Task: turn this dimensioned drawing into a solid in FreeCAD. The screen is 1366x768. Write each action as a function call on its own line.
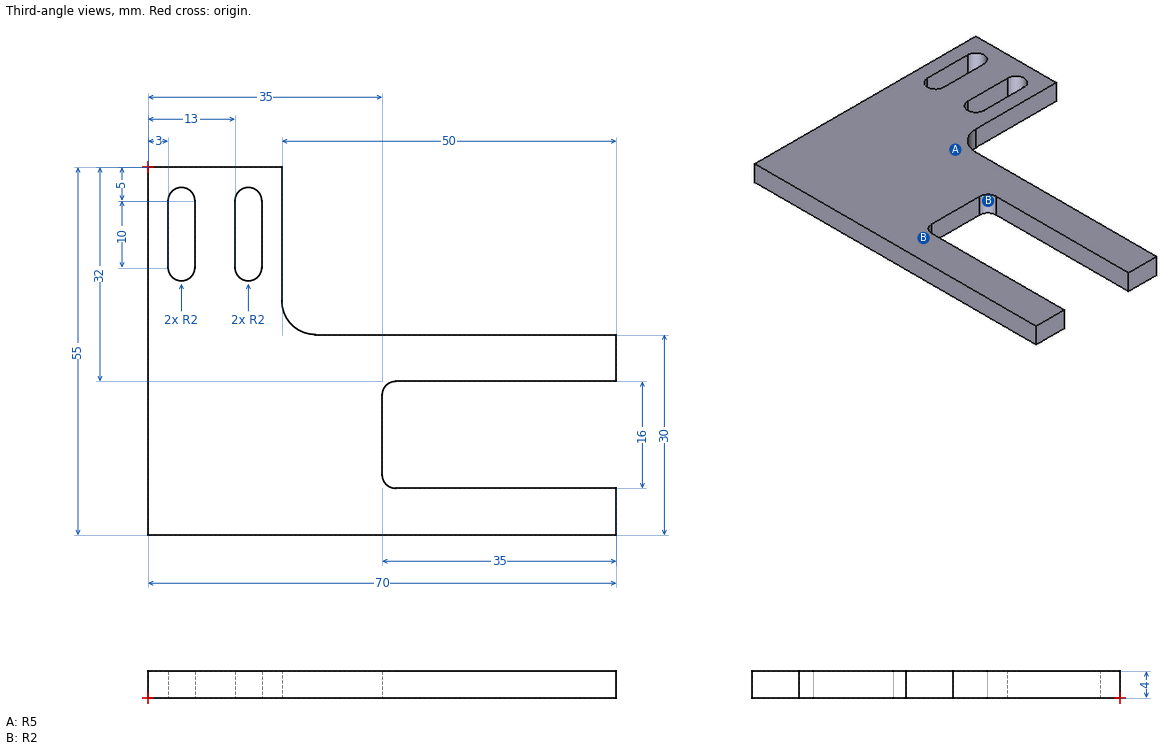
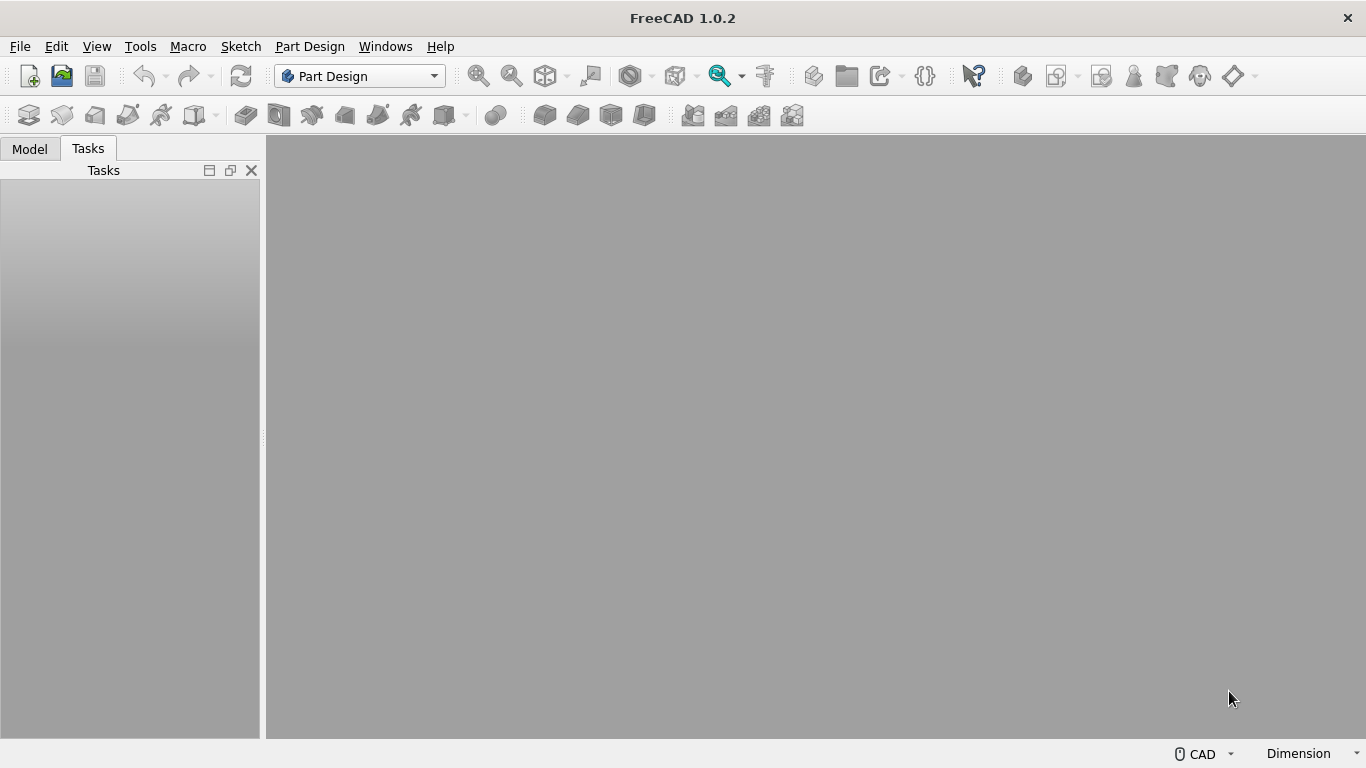
click(29, 76)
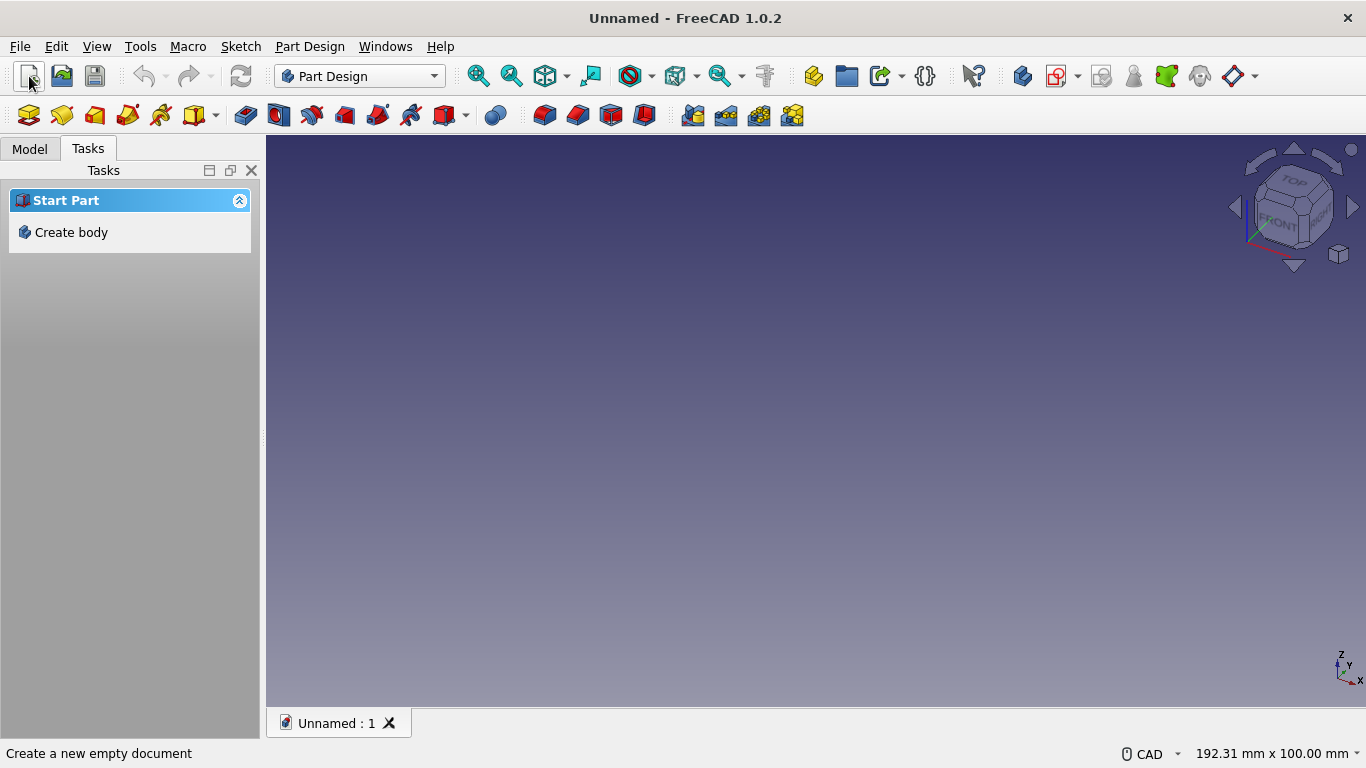
click(1056, 76)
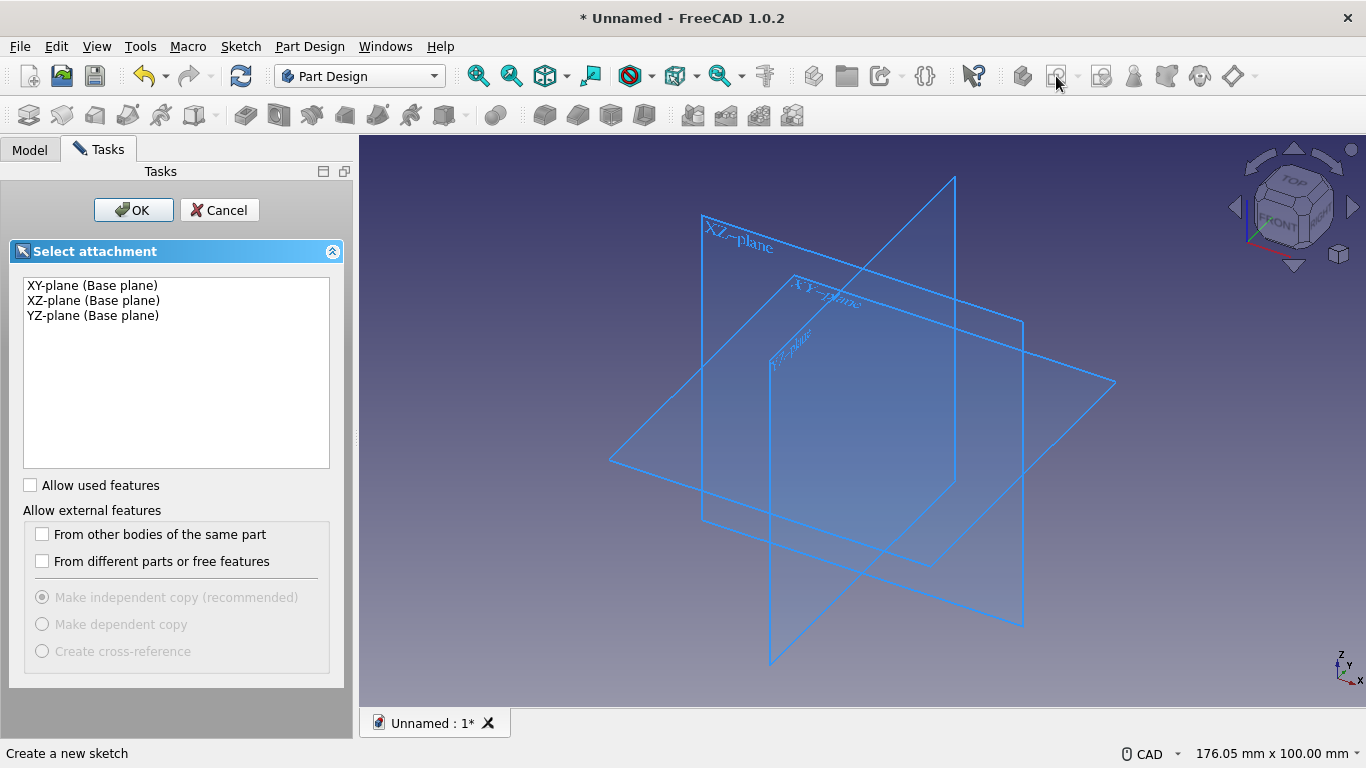
click(84, 286)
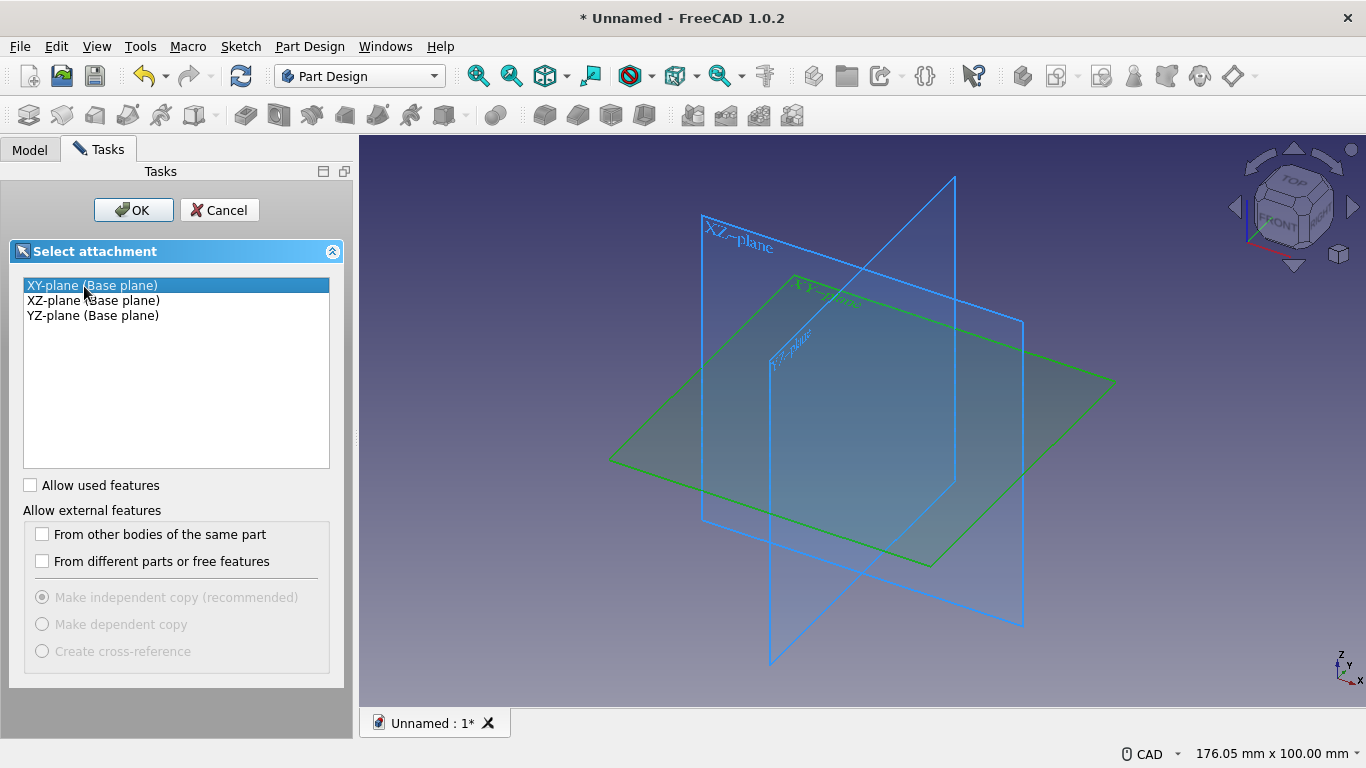
click(134, 210)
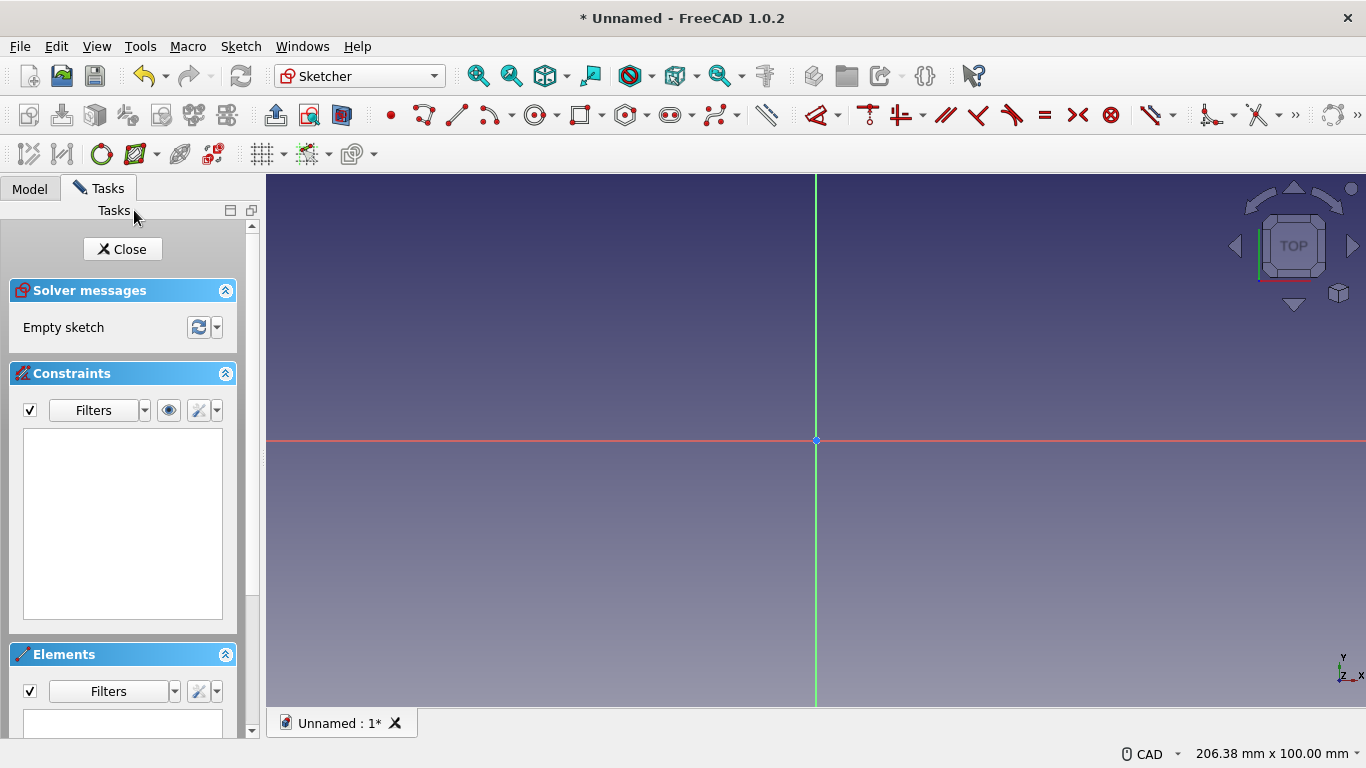
scroll(294, 202, down, 1)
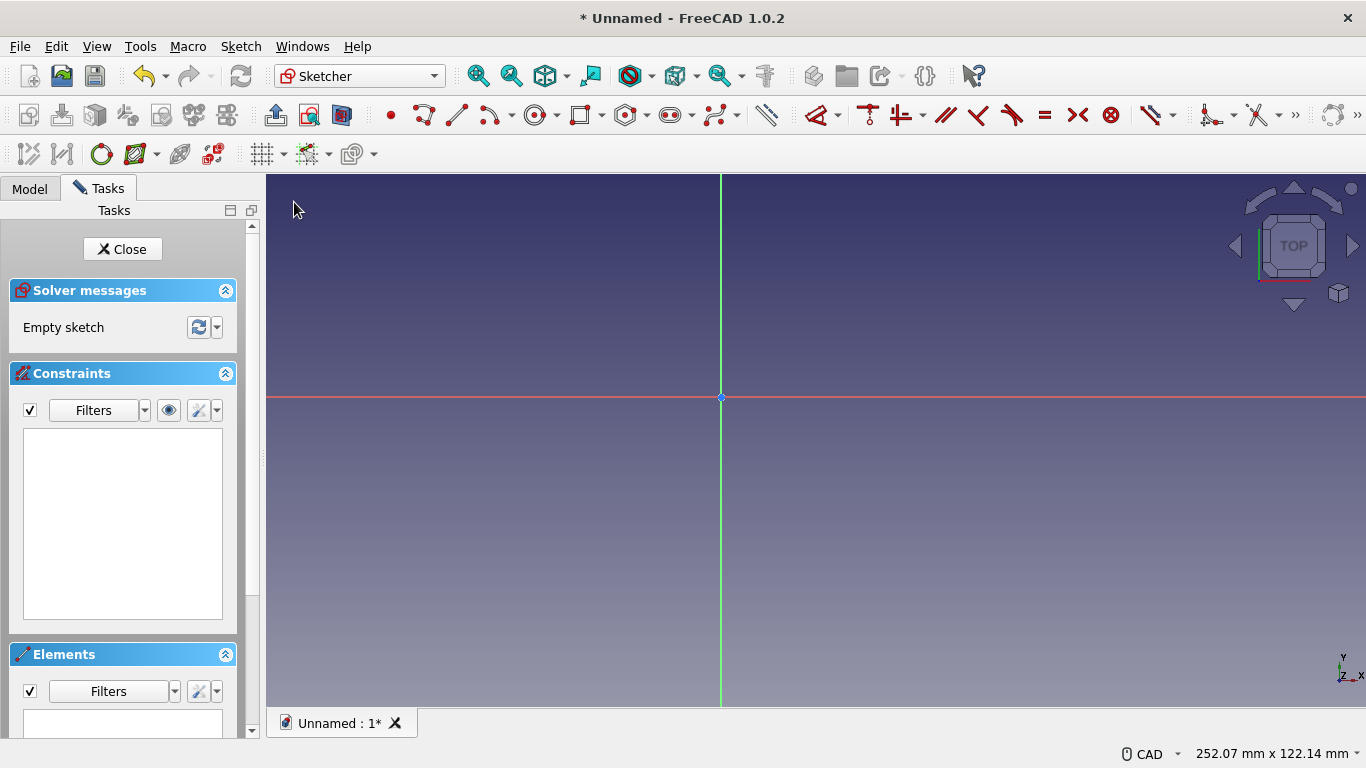
scroll(1132, 673, up, 2)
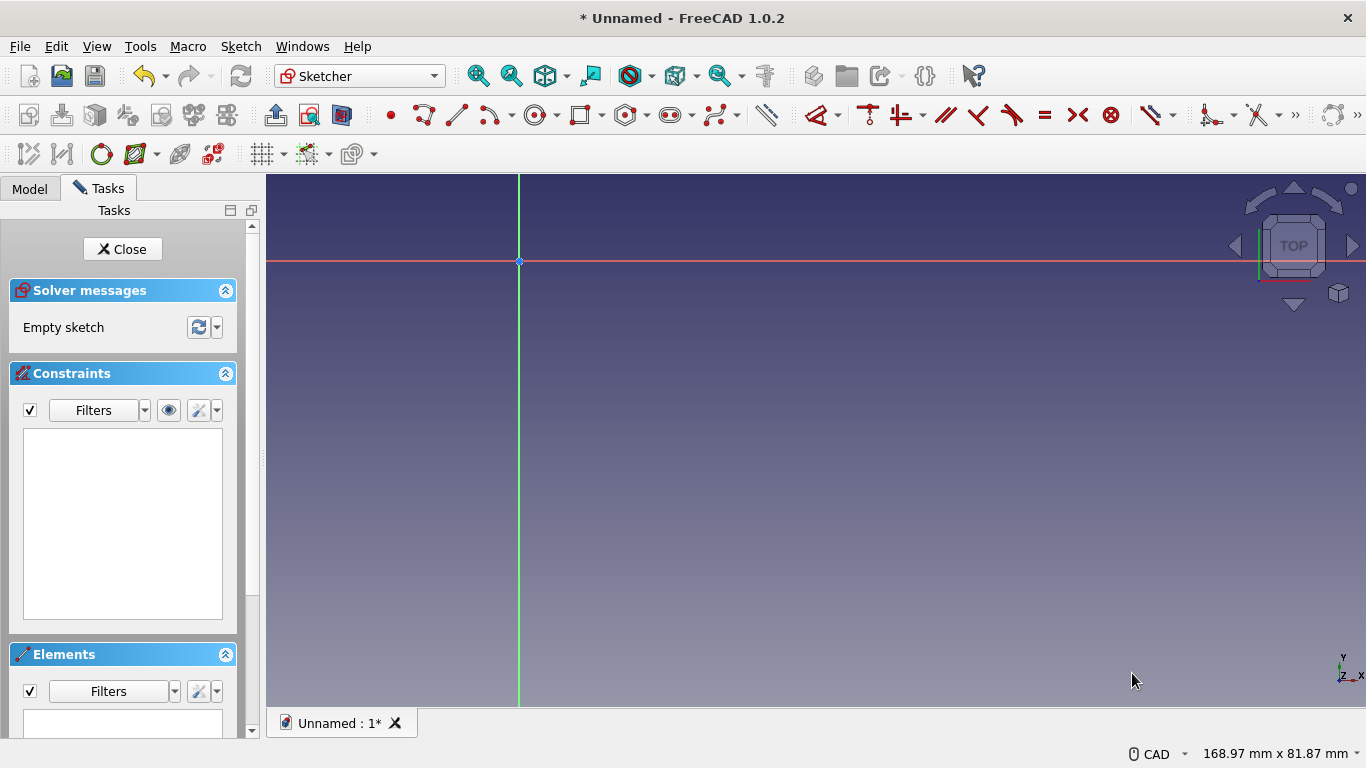
key(g)
key(m)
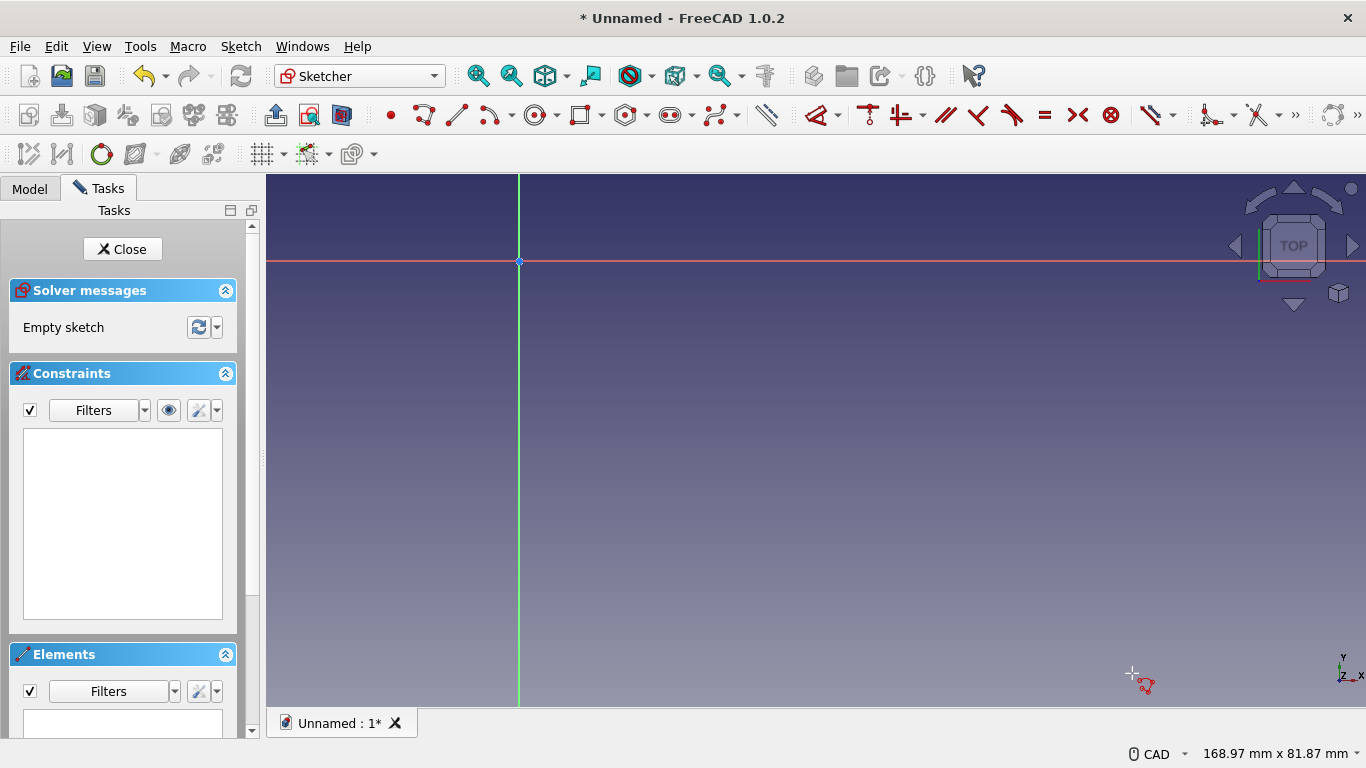
click(519, 261)
click(528, 619)
click(975, 619)
click(975, 424)
click(649, 424)
click(649, 270)
click(519, 261)
key(Escape)
key(Escape)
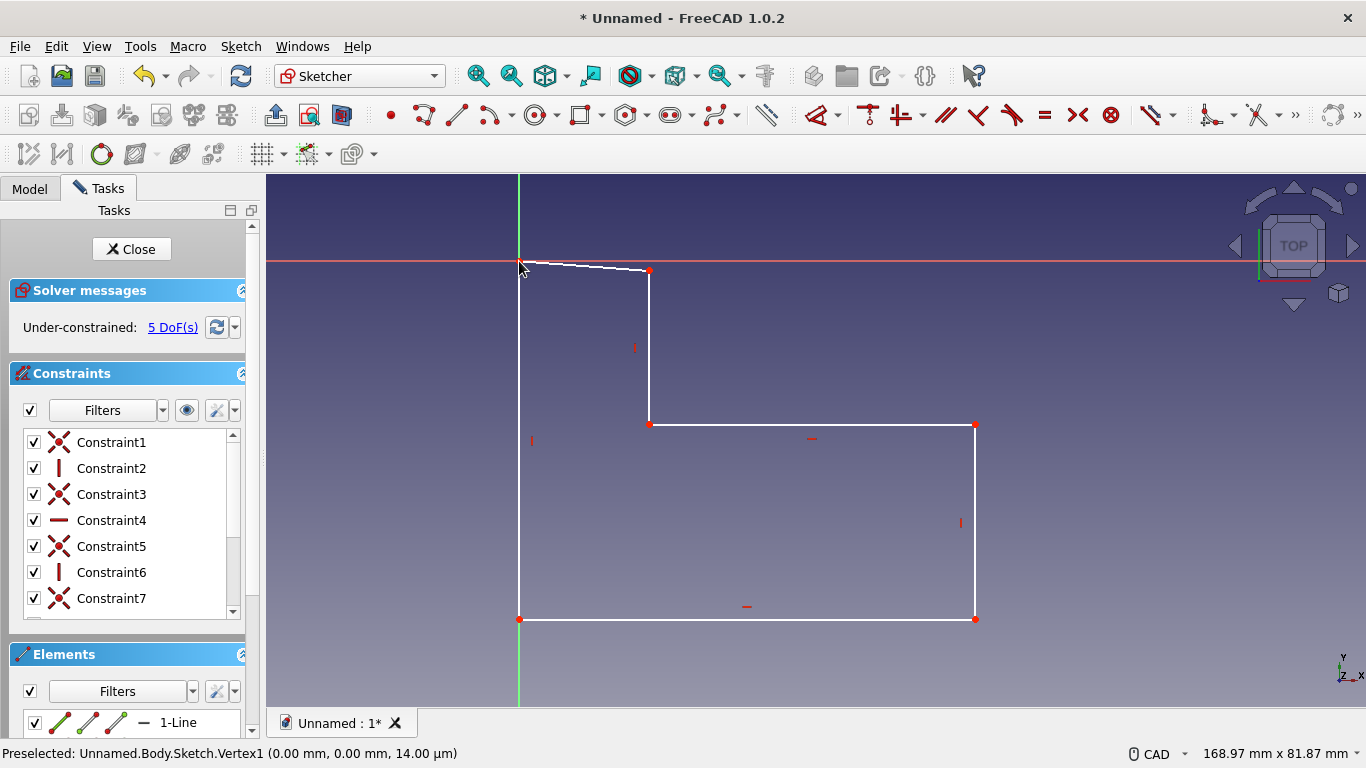
click(558, 264)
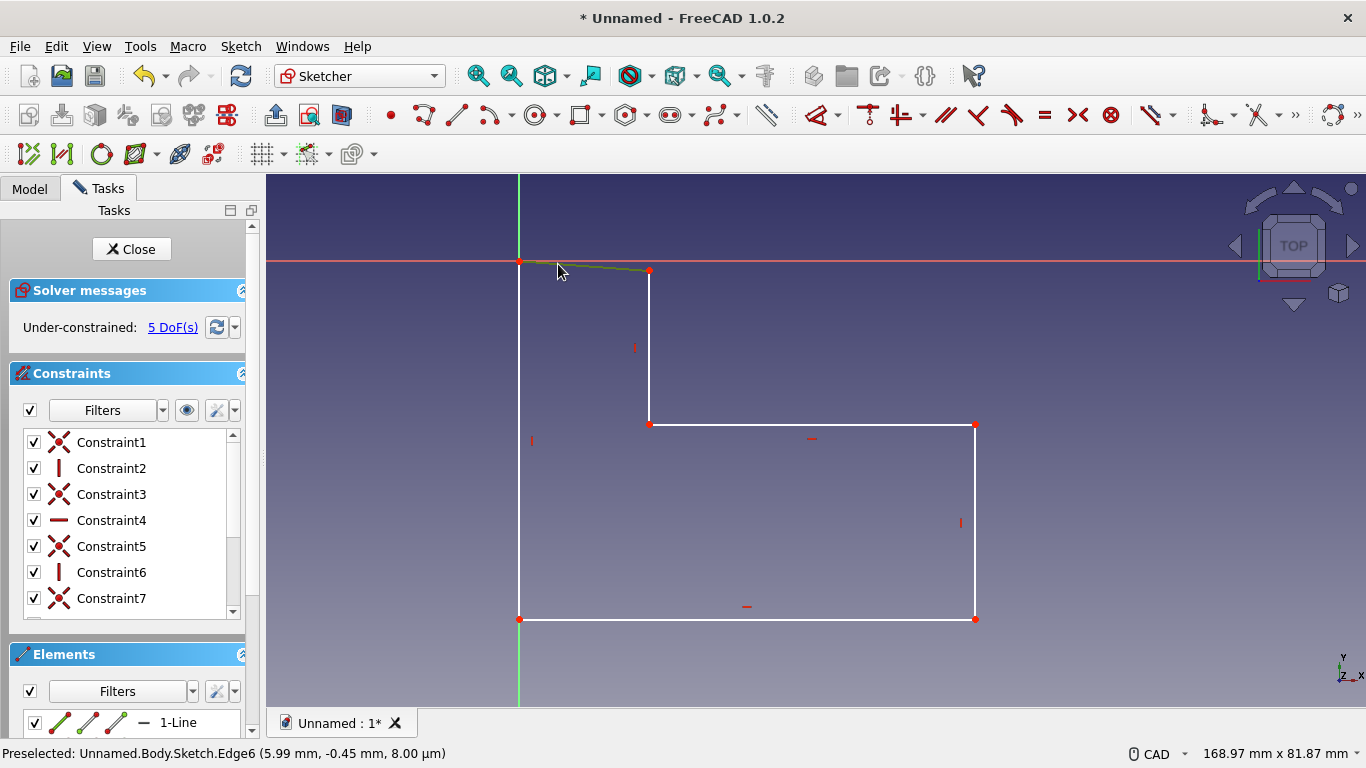
click(922, 116)